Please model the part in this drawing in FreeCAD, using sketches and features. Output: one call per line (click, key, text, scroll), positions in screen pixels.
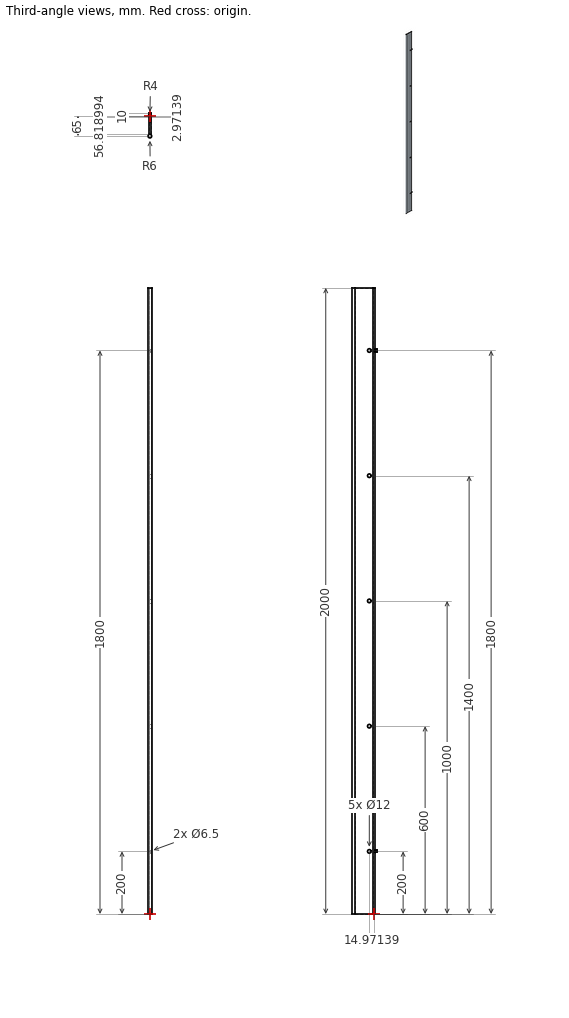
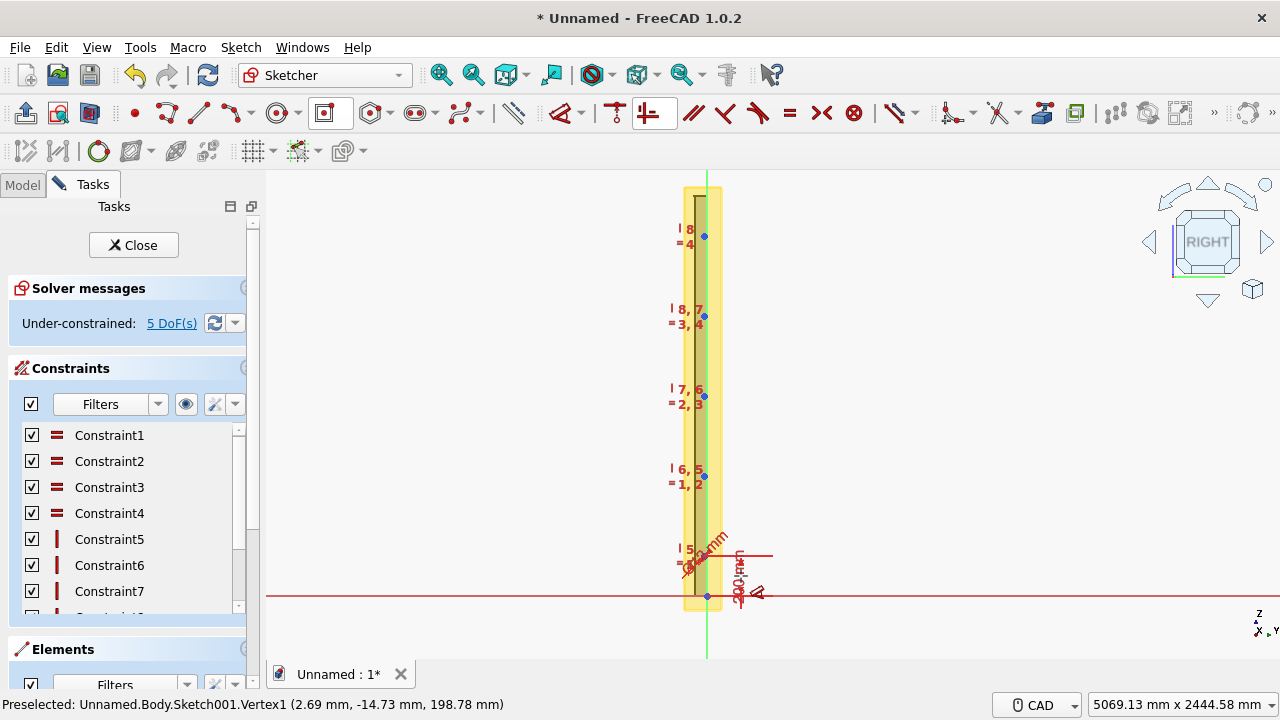
click(704, 476)
click(741, 509)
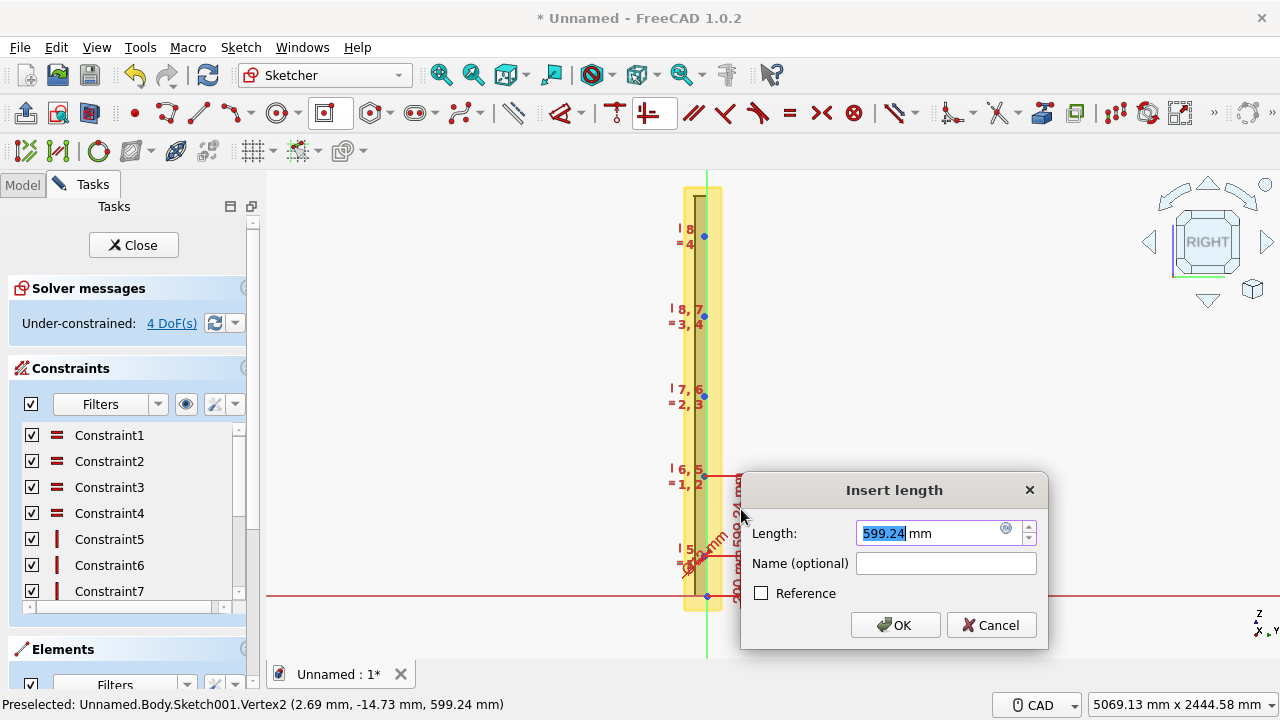
text(600)
key(Return)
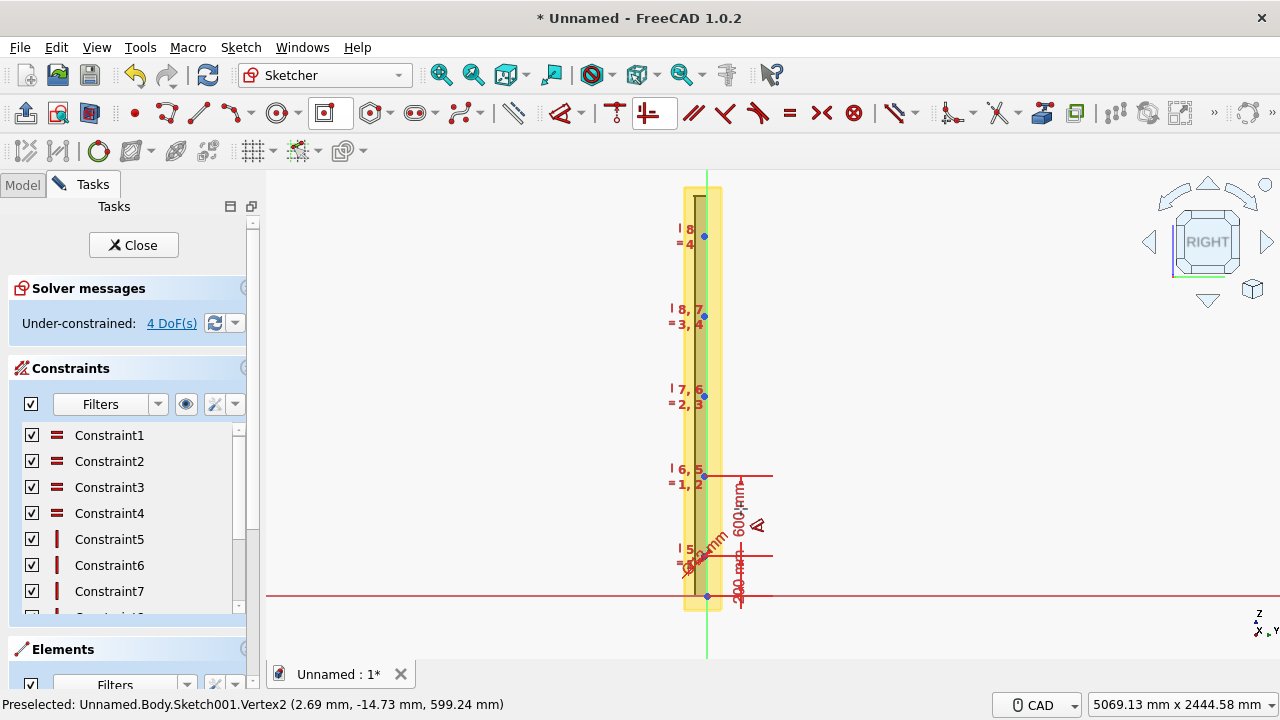
click(704, 396)
click(741, 450)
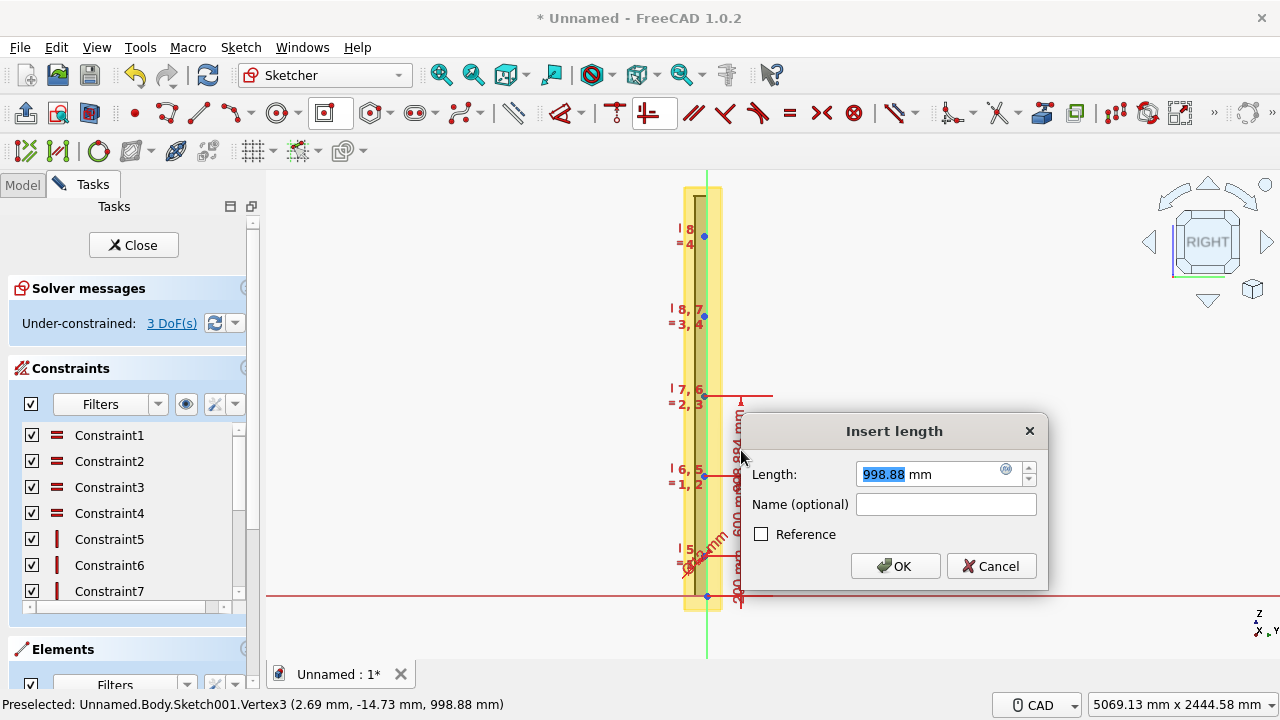
text(1000)
key(Return)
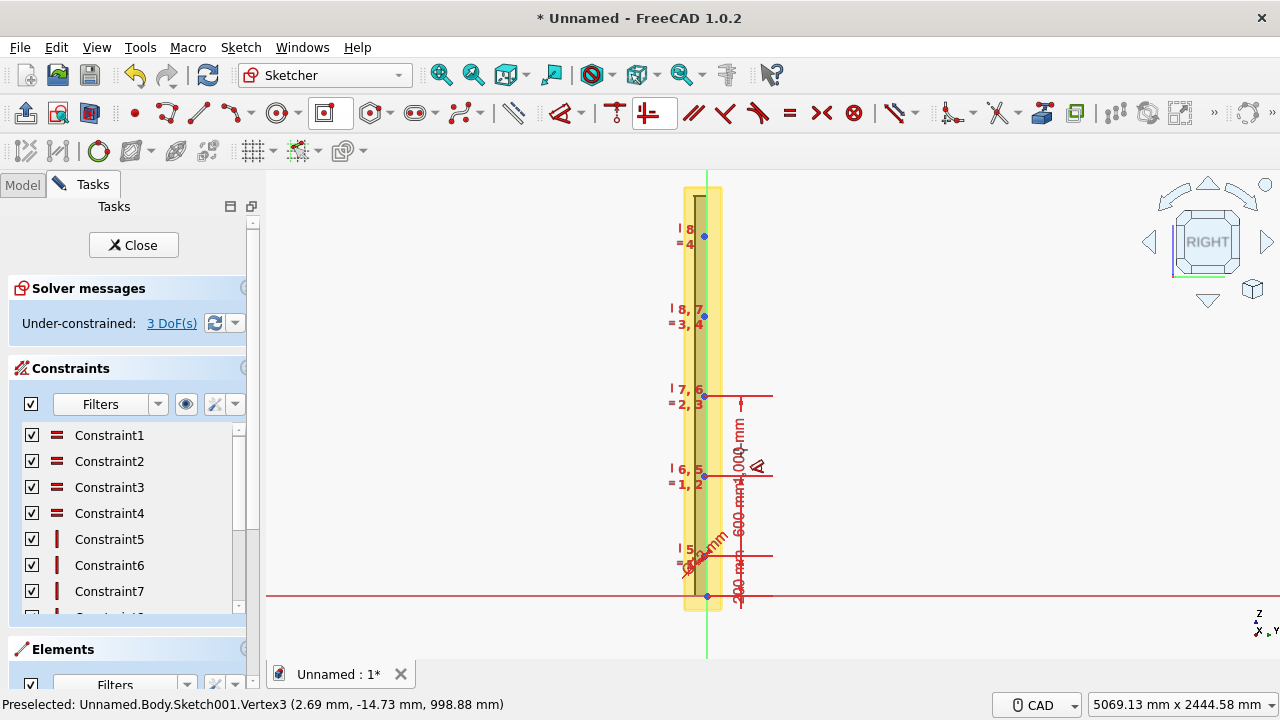
click(704, 316)
click(741, 392)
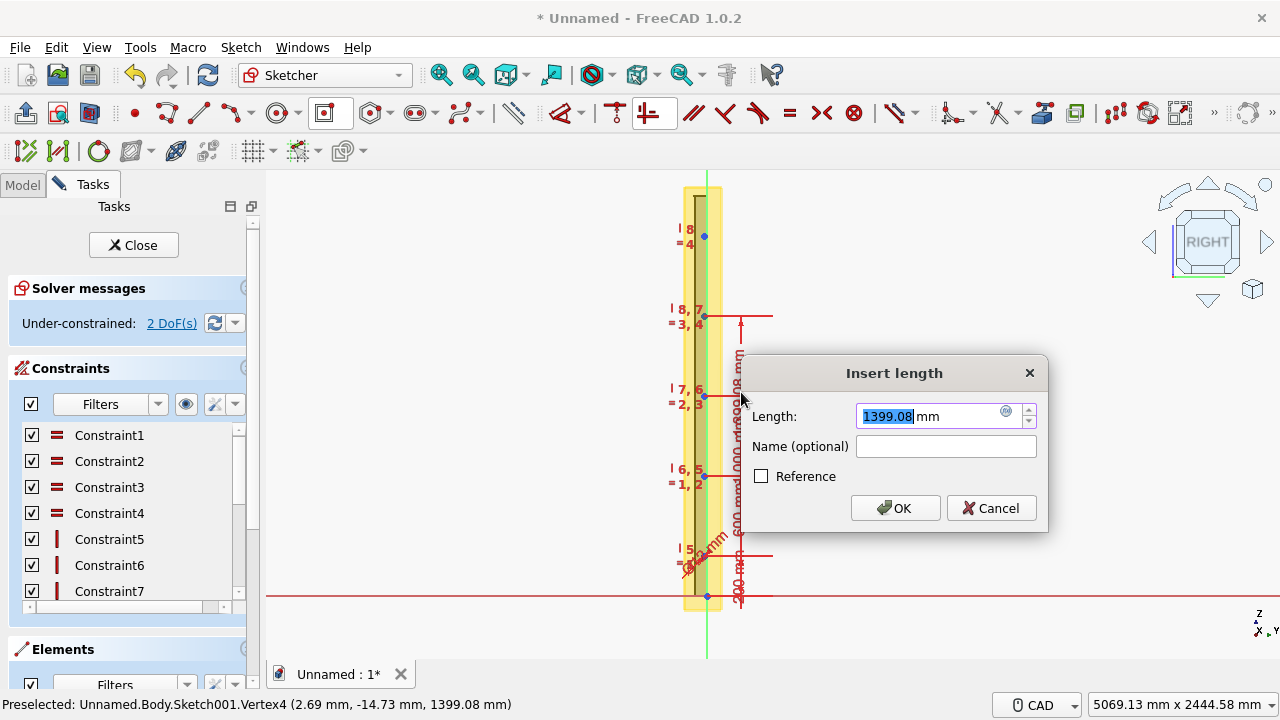
text(1400)
key(Return)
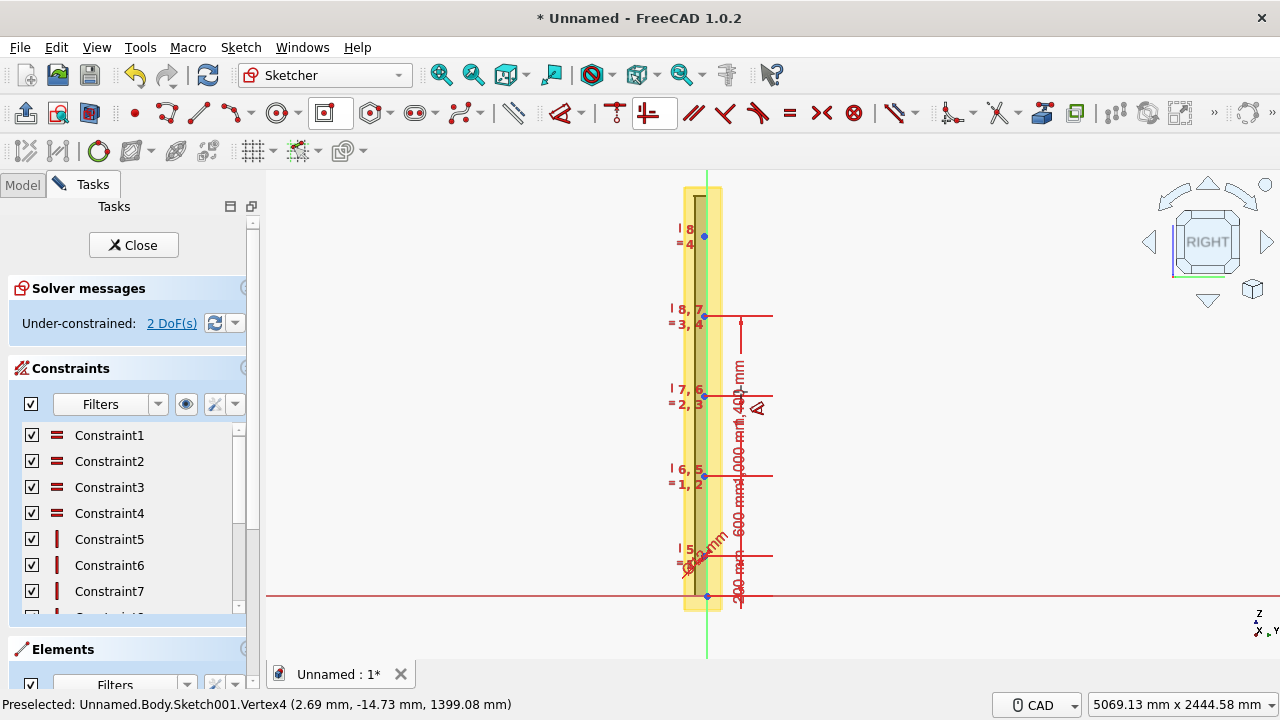
click(704, 236)
click(741, 416)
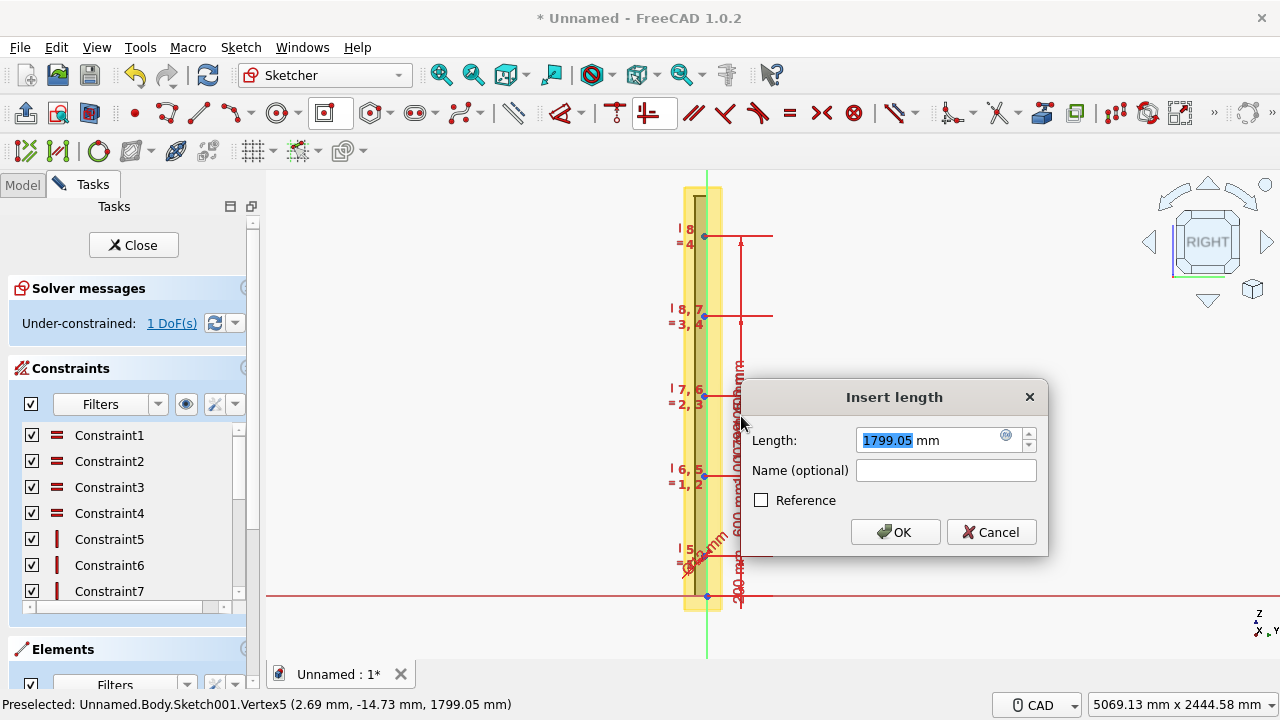
text(1800)
key(Return)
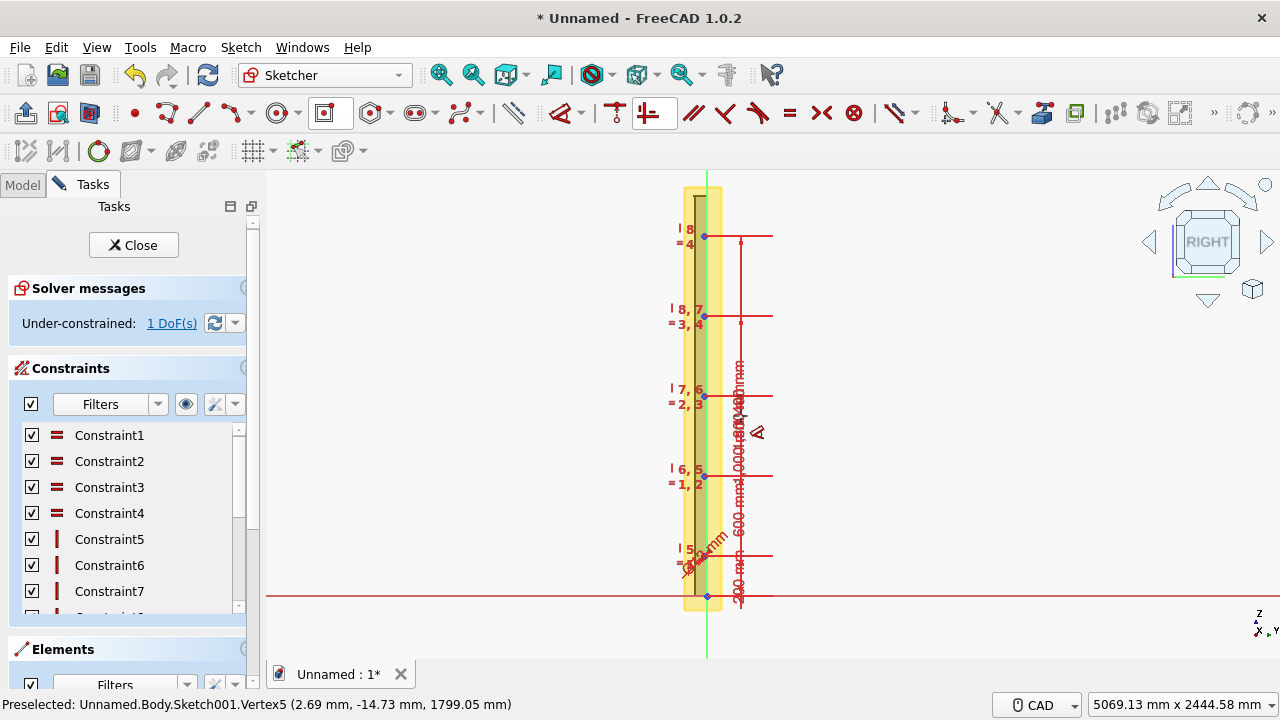
scroll(704, 556, up, 13)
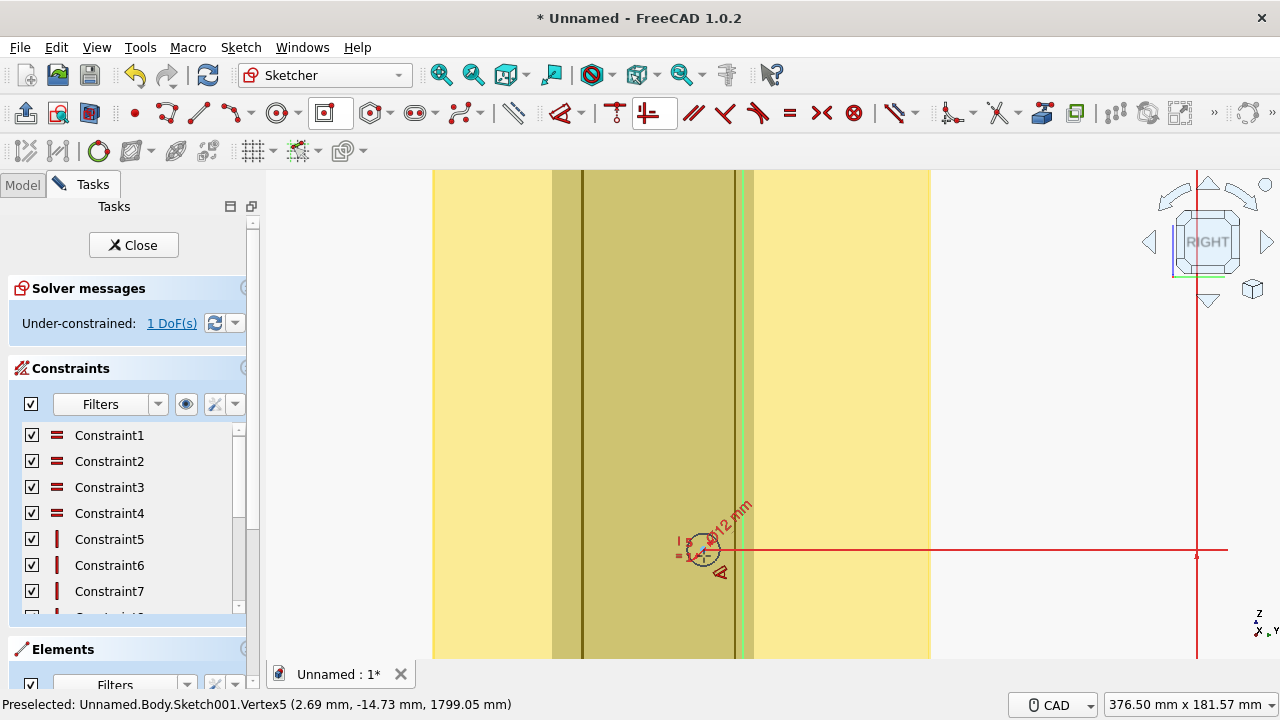
click(704, 550)
click(723, 492)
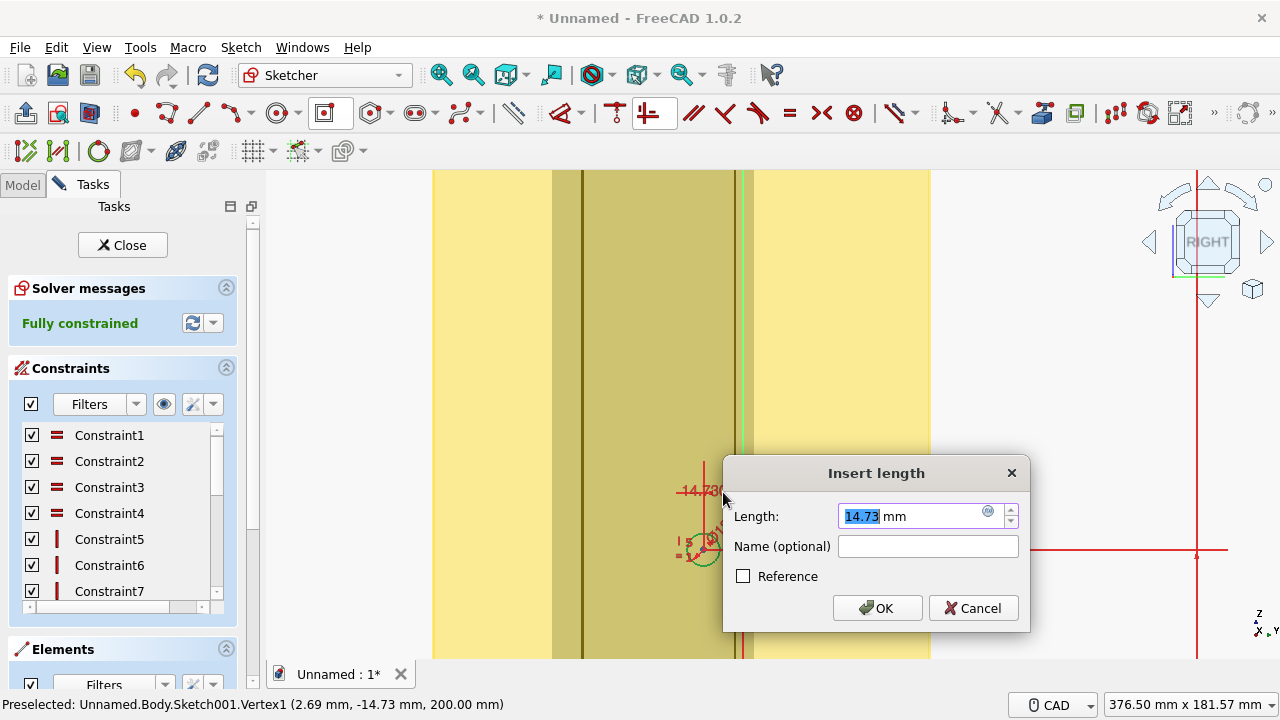
text(14.97139)
key(Return)
key(Escape)